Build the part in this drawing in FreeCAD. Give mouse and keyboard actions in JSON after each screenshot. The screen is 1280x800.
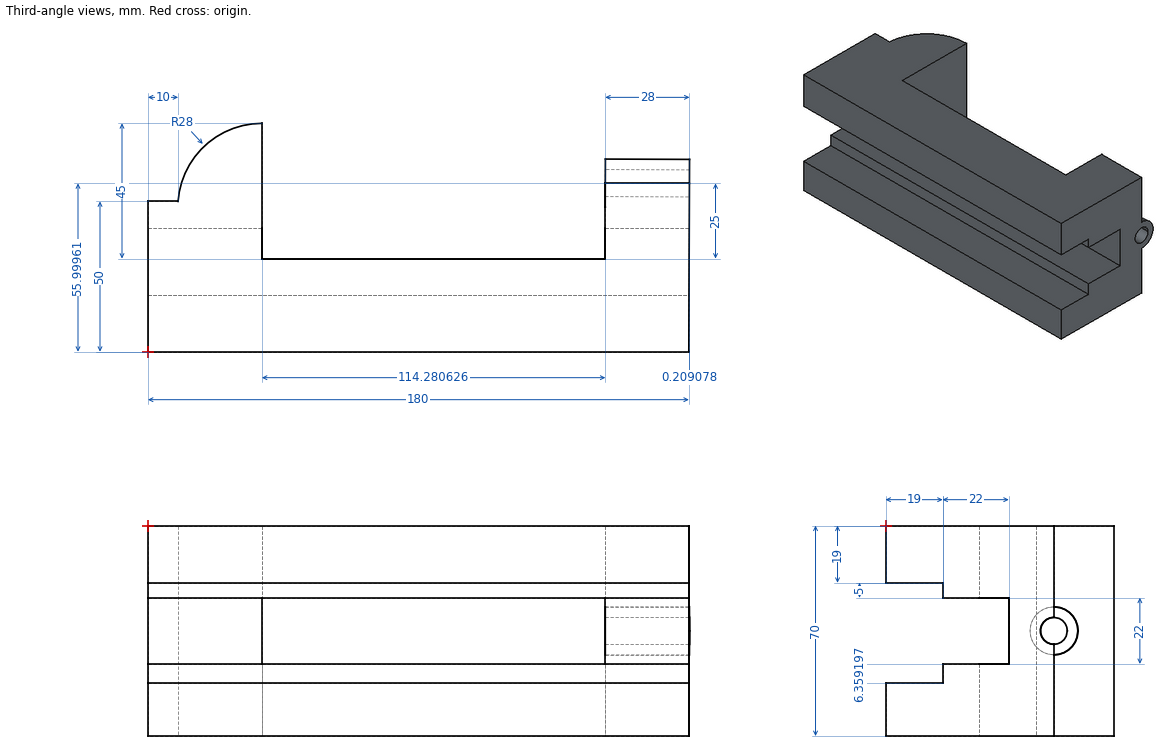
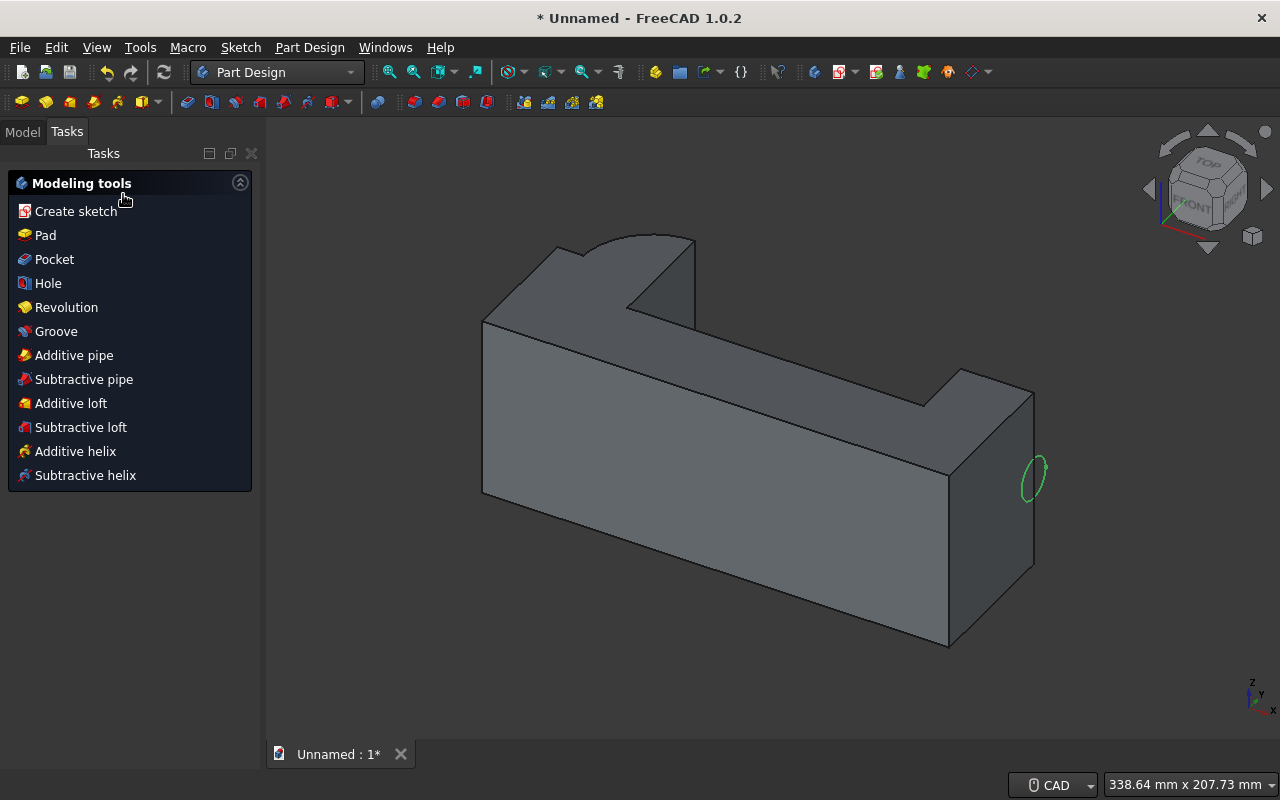
{"action": "left_click", "coordinate": [22, 102]}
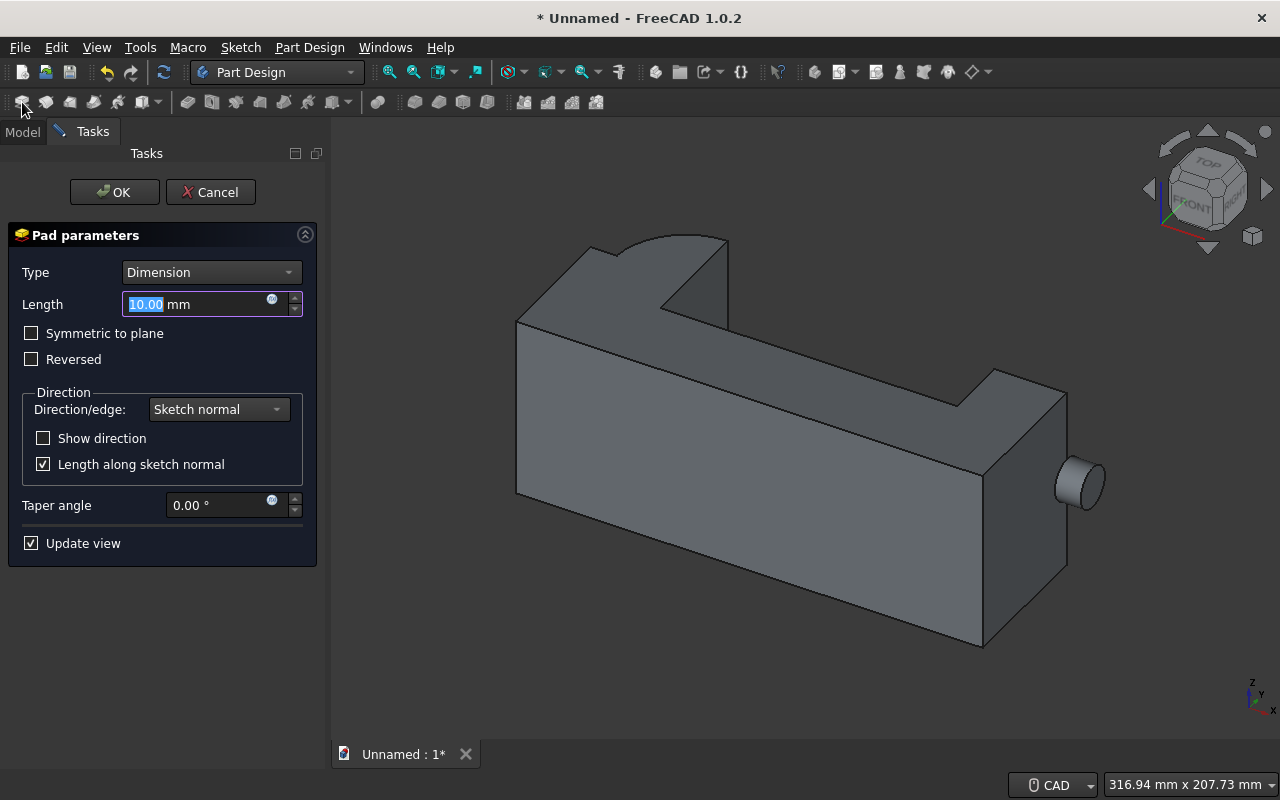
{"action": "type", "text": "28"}
{"action": "key", "text": "Tab"}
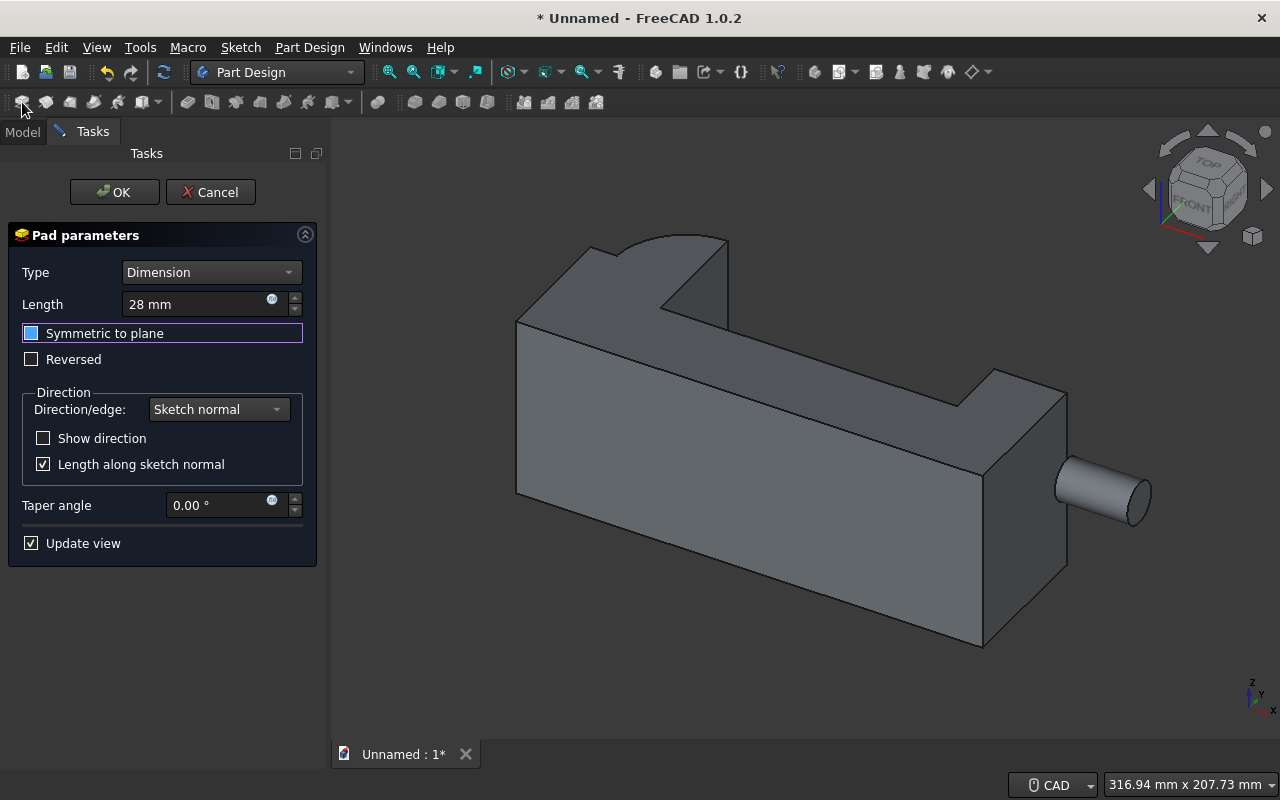
{"action": "left_click", "coordinate": [30, 359]}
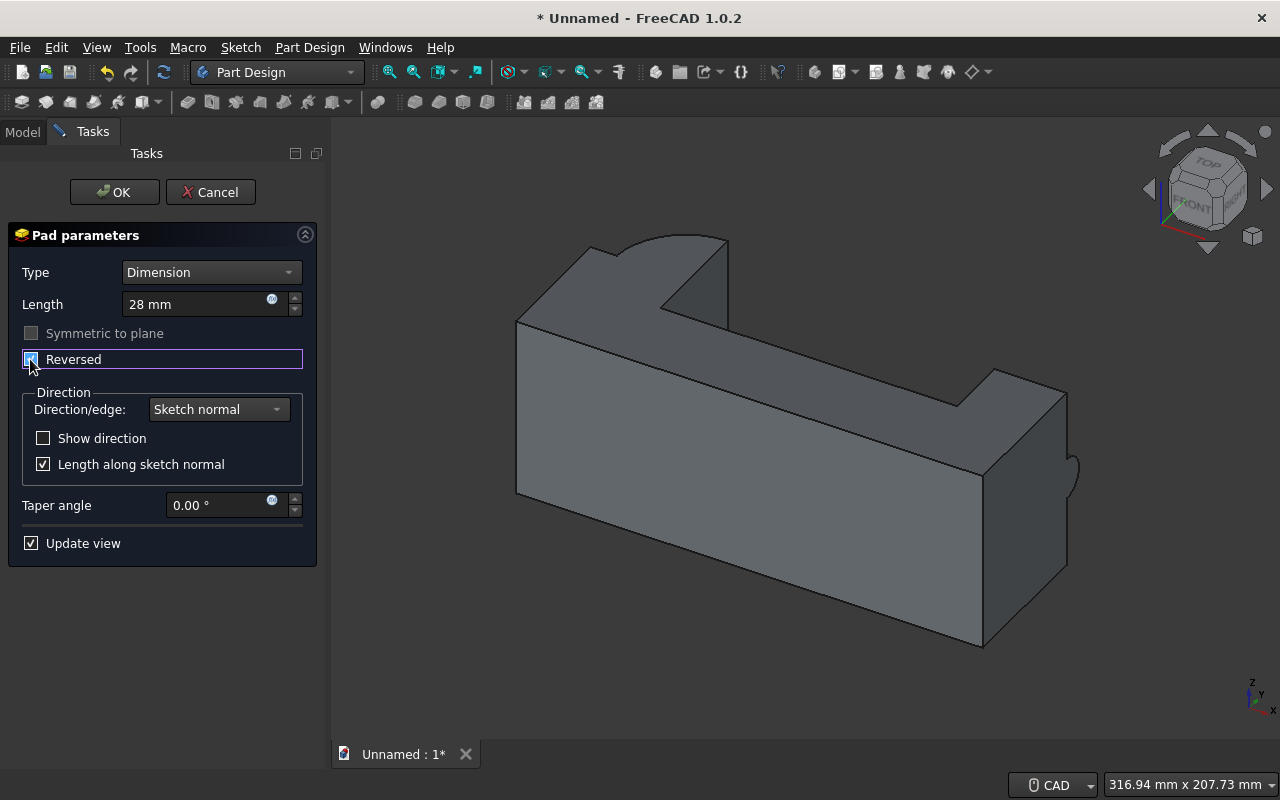
{"action": "left_click", "coordinate": [115, 192]}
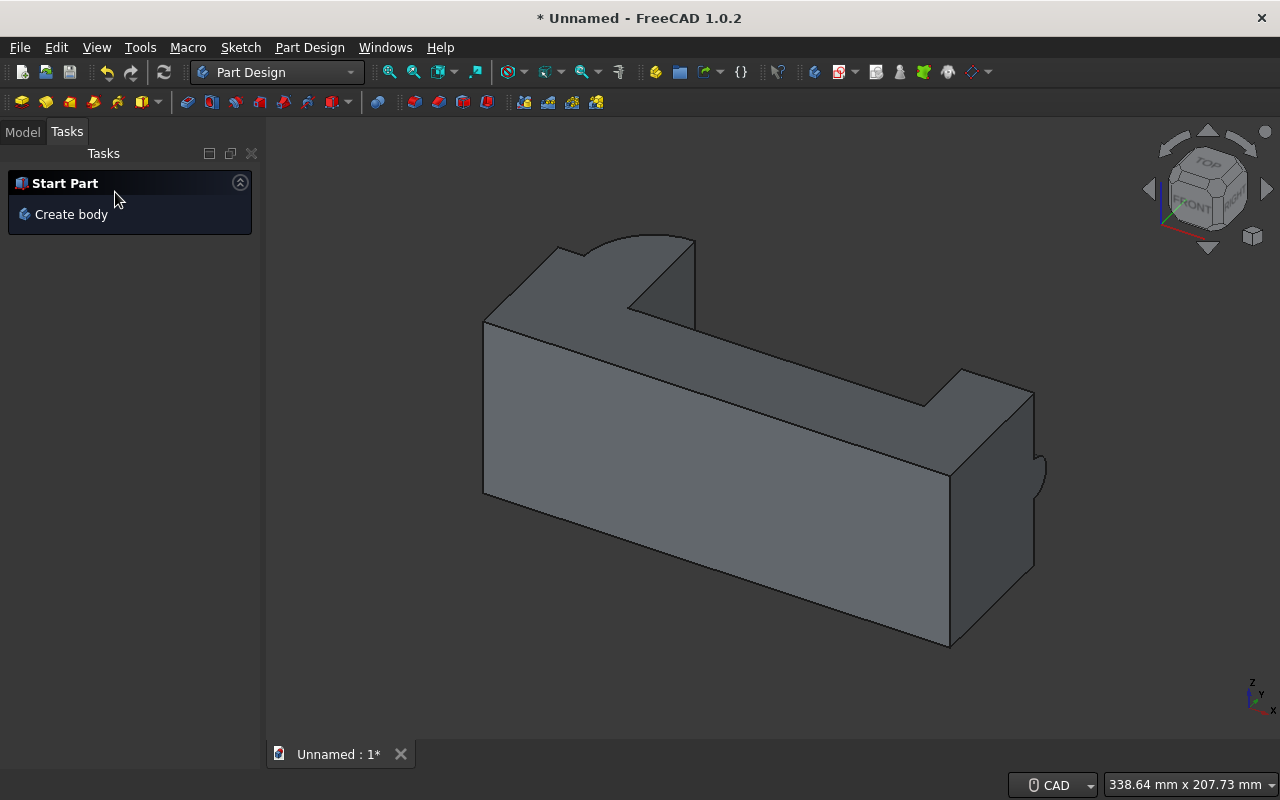
{"action": "left_click", "coordinate": [998, 513]}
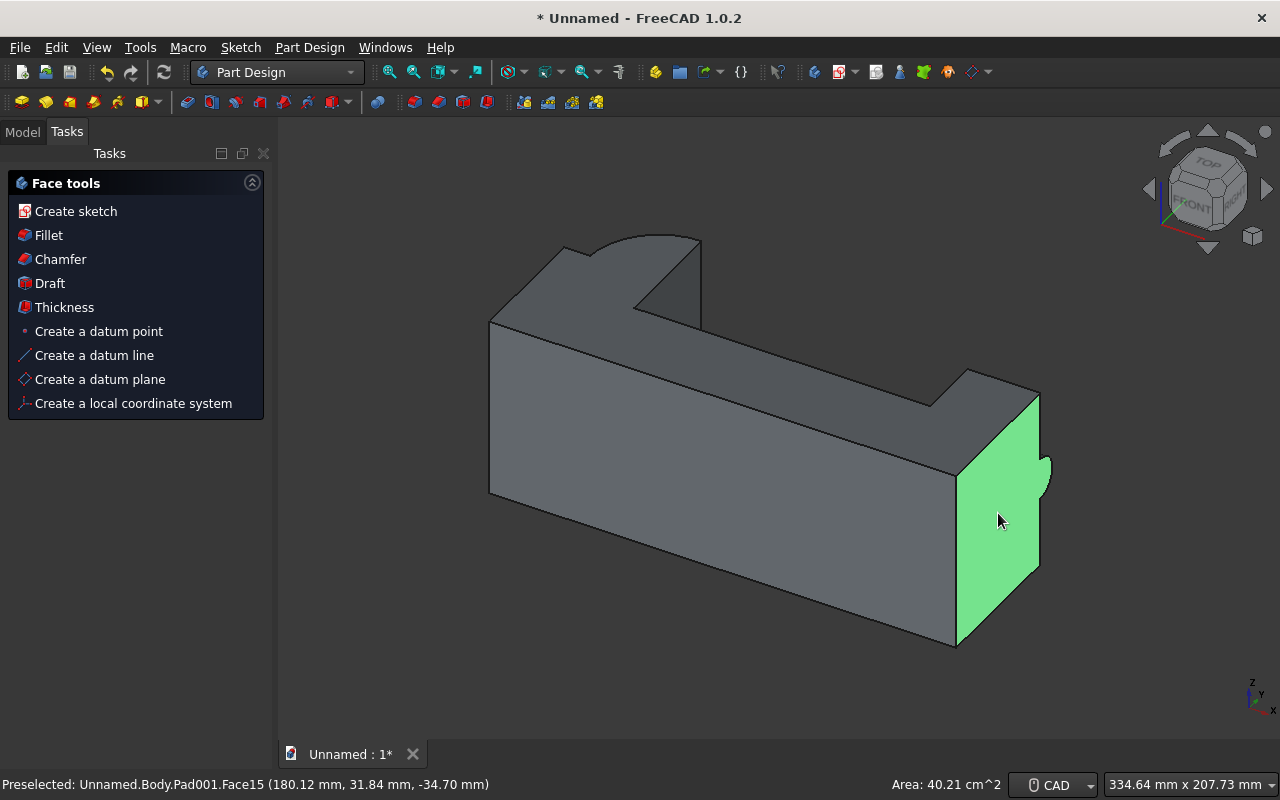
{"action": "left_click", "coordinate": [840, 72]}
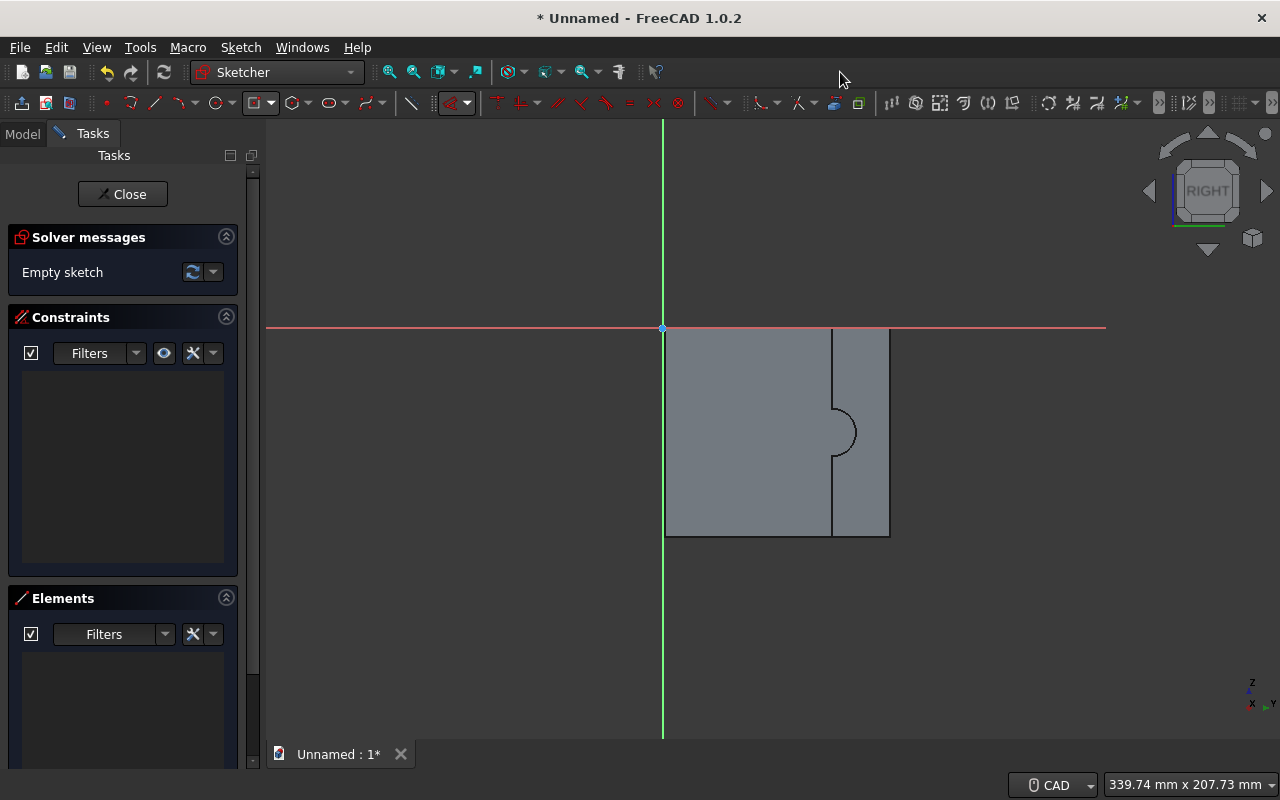
{"action": "left_click", "coordinate": [70, 104]}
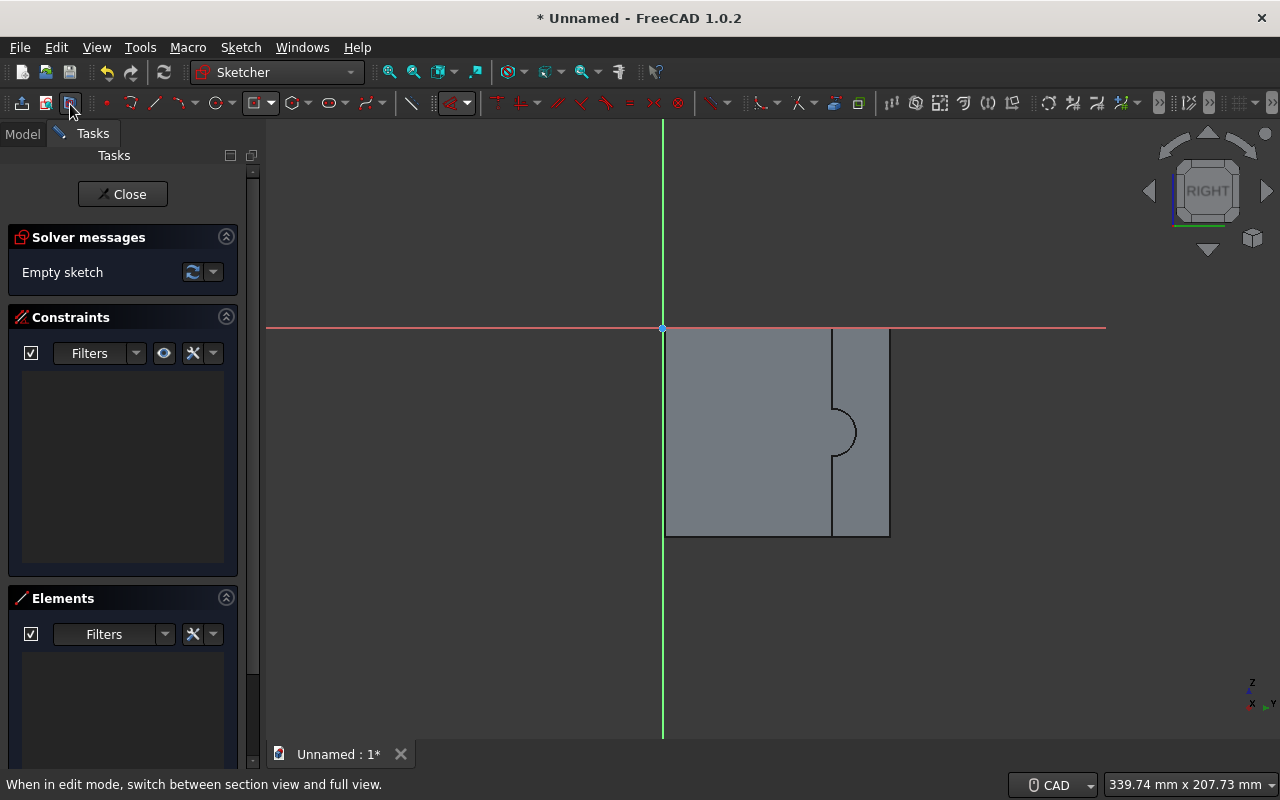
{"action": "scroll", "coordinate": [842, 433], "scroll_direction": "up", "scroll_amount": 13}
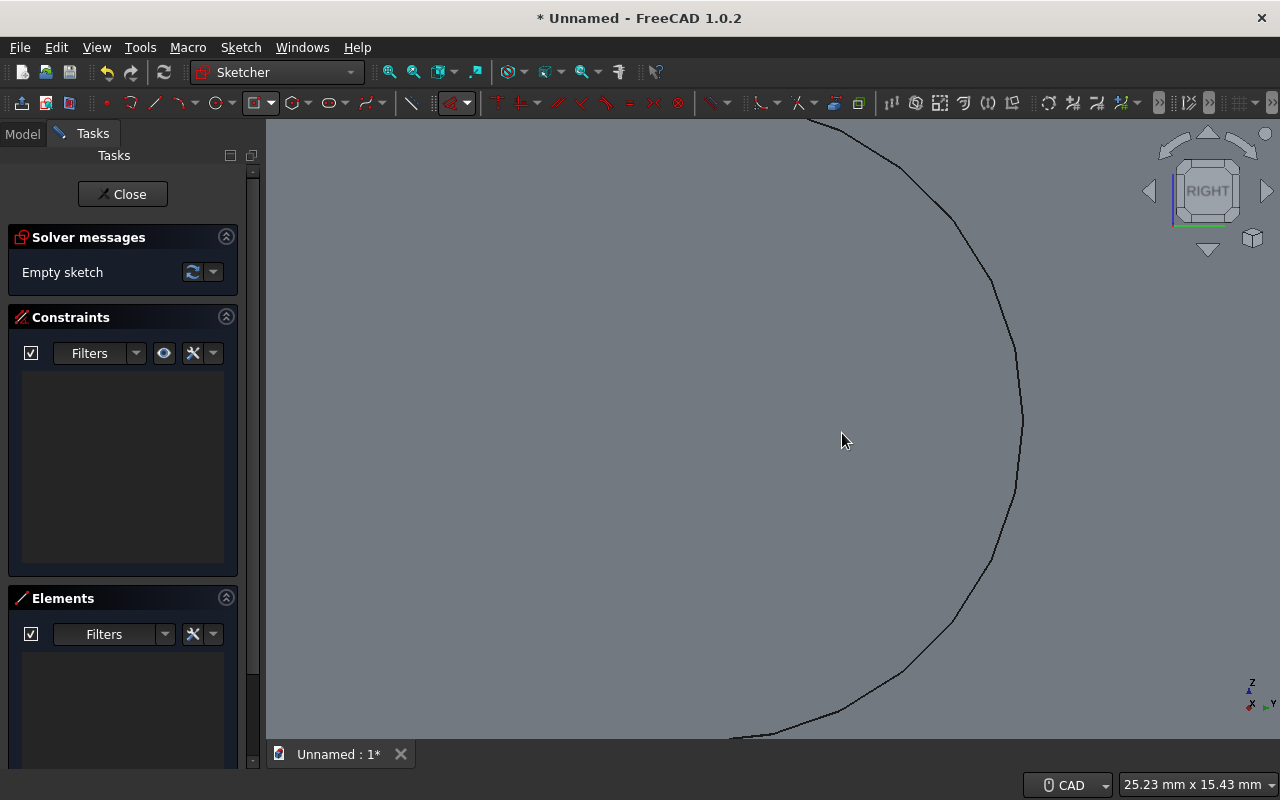
{"action": "left_click", "coordinate": [216, 104]}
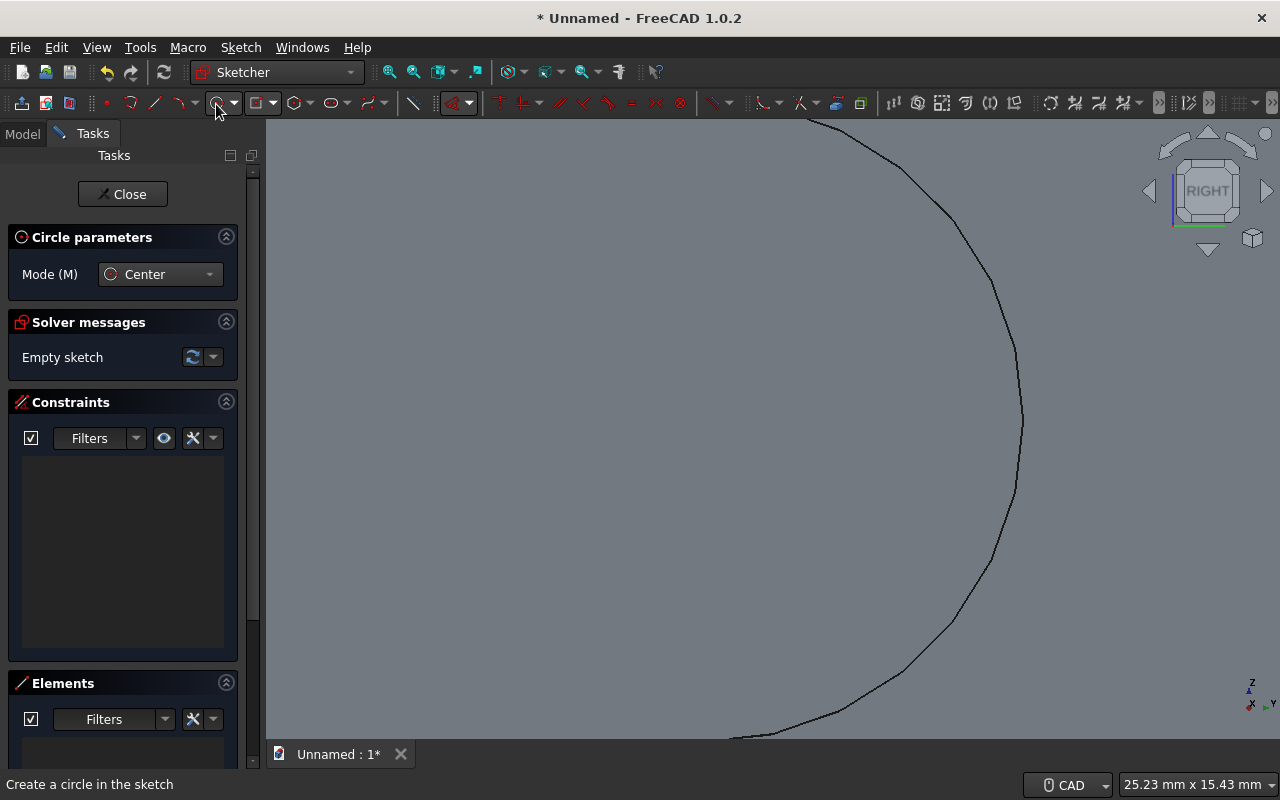
{"action": "left_click", "coordinate": [702, 421]}
{"action": "mouse_move", "coordinate": [830, 293]}